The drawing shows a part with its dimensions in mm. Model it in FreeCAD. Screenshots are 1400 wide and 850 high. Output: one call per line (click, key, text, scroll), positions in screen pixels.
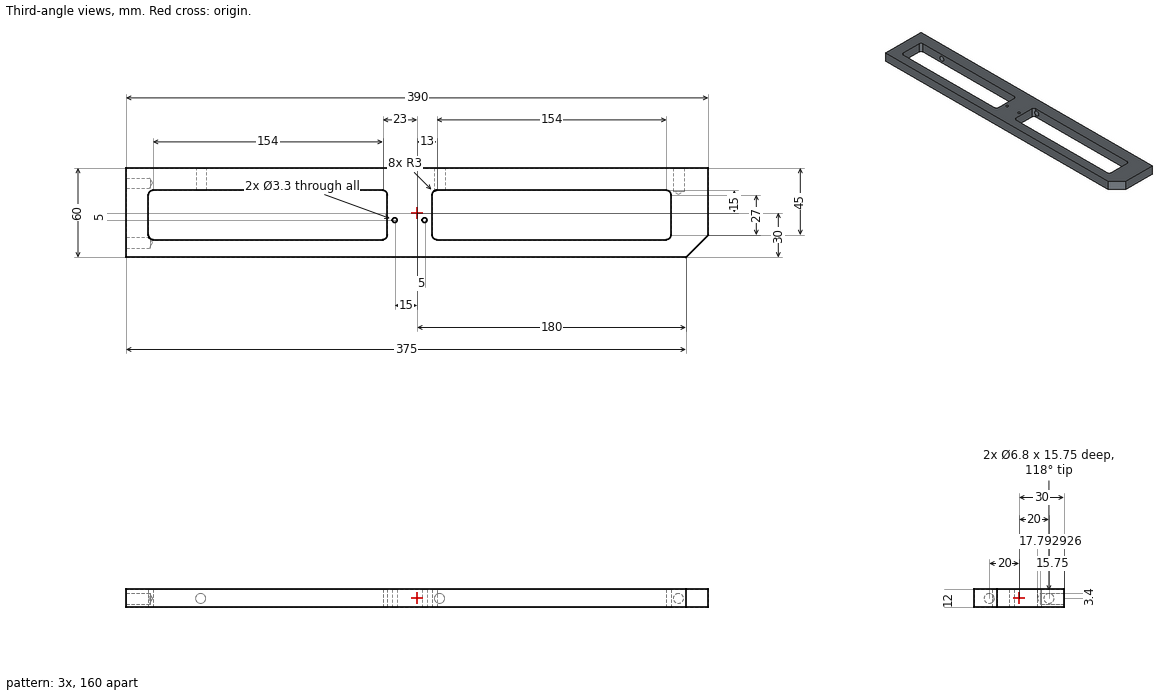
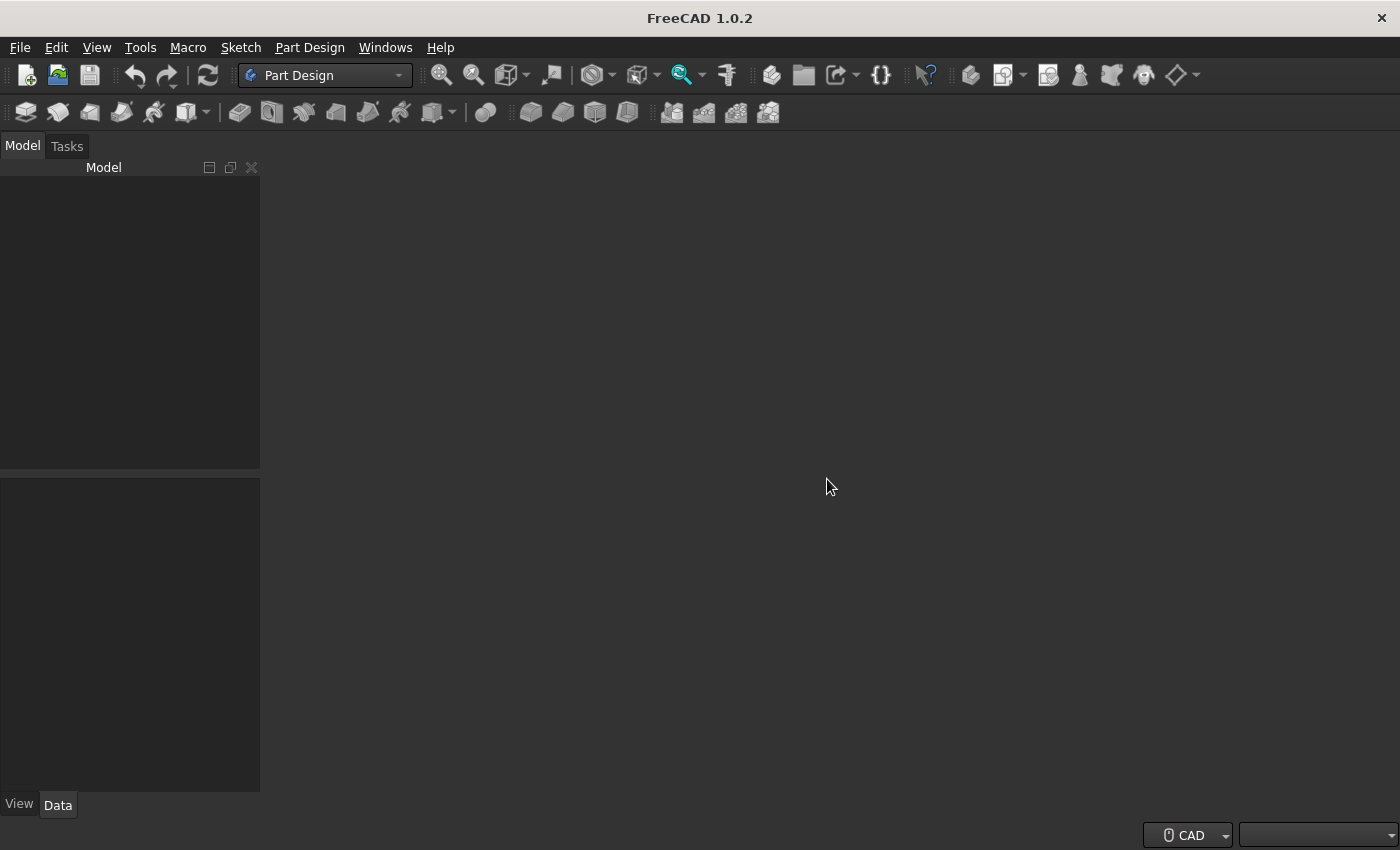
click(26, 76)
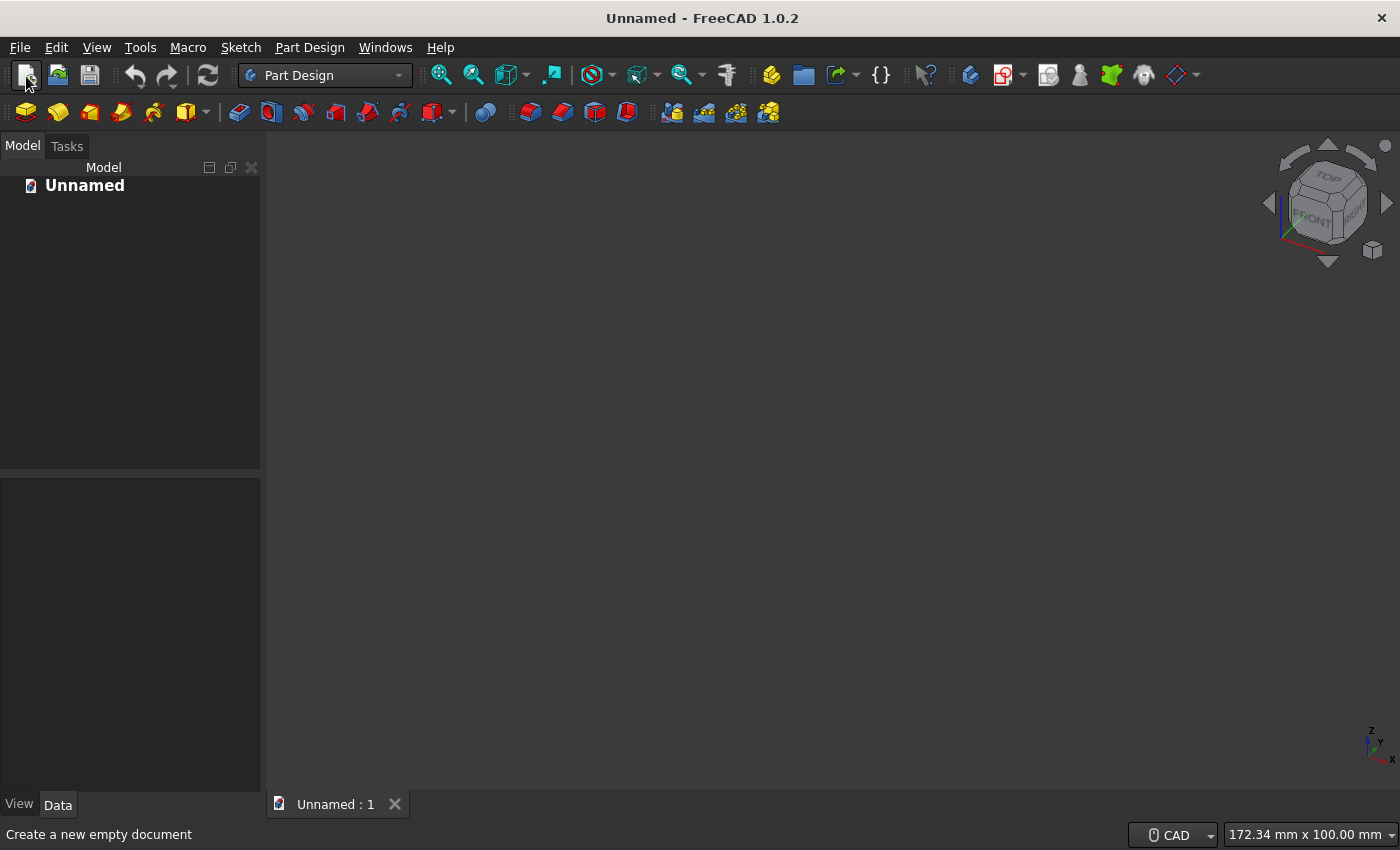
click(1004, 76)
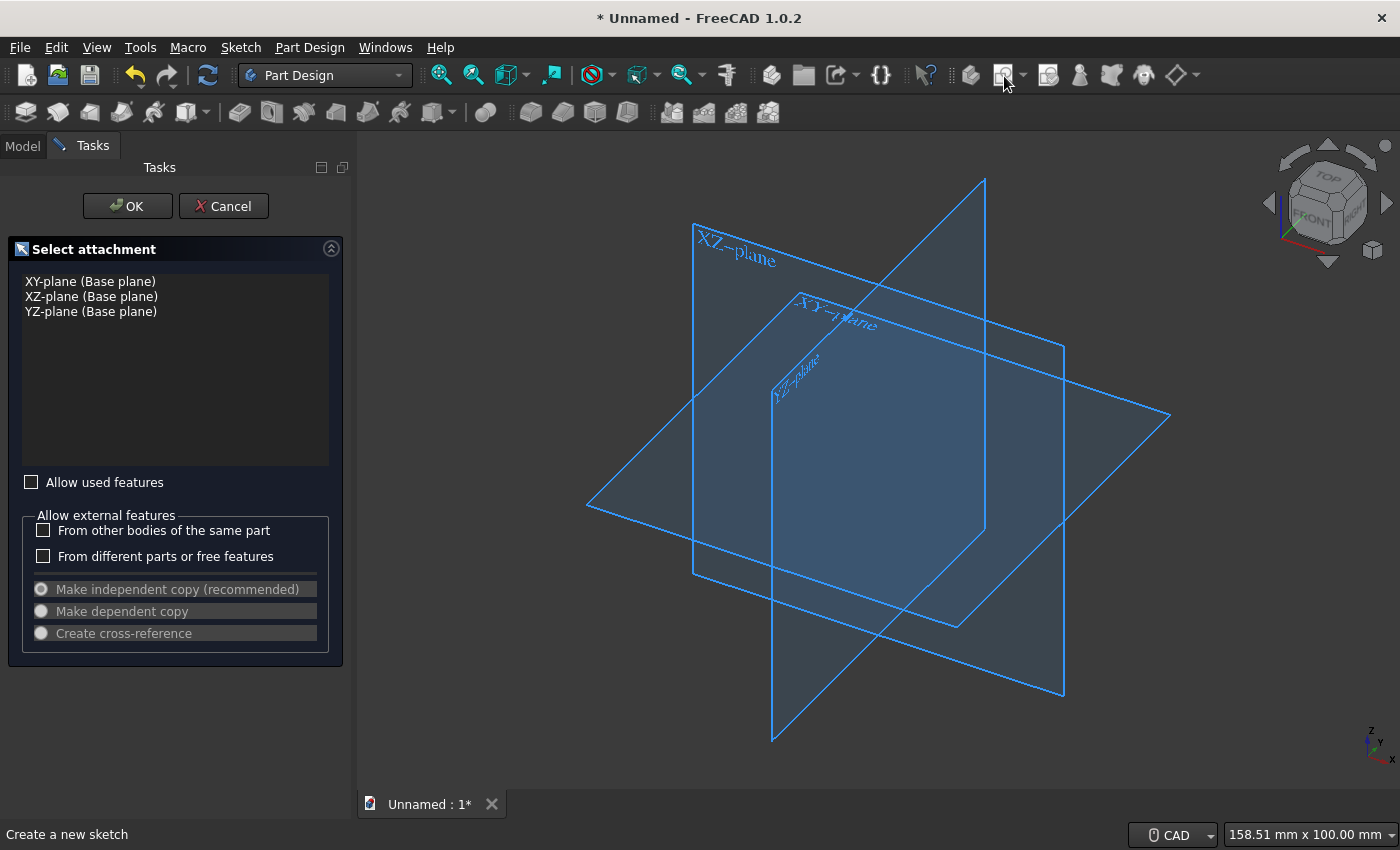
click(82, 282)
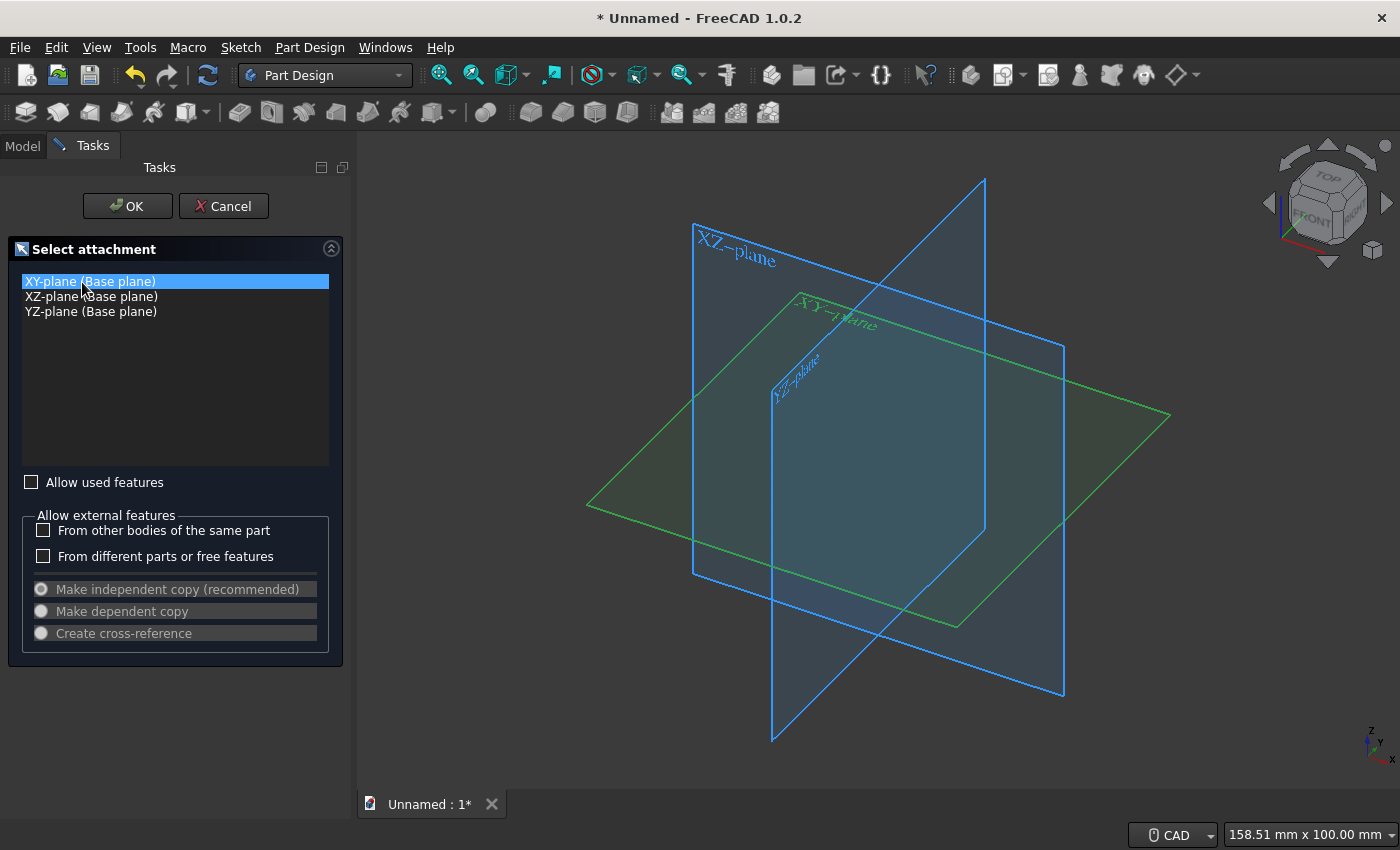
click(128, 206)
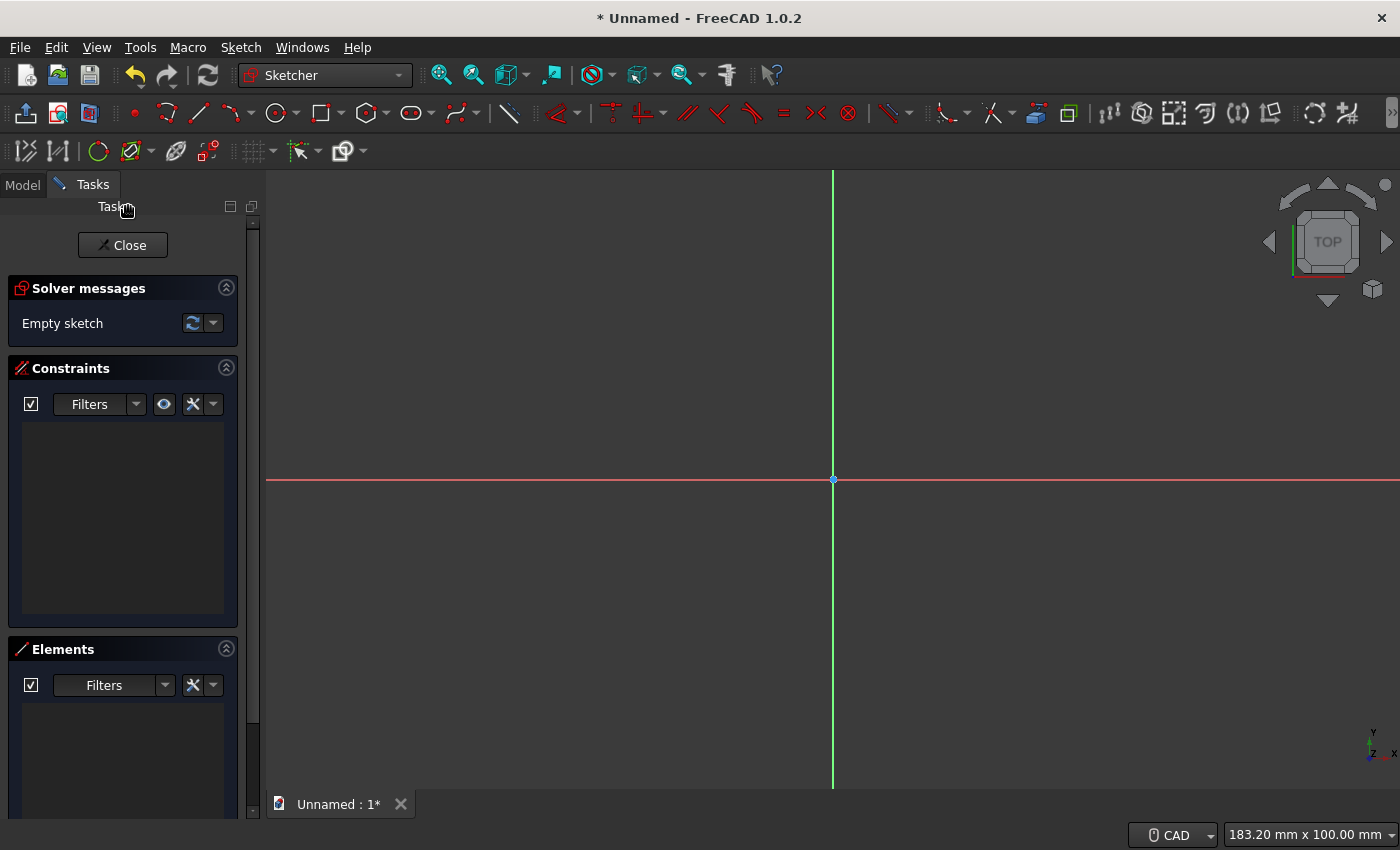
scroll(735, 480, down, 6)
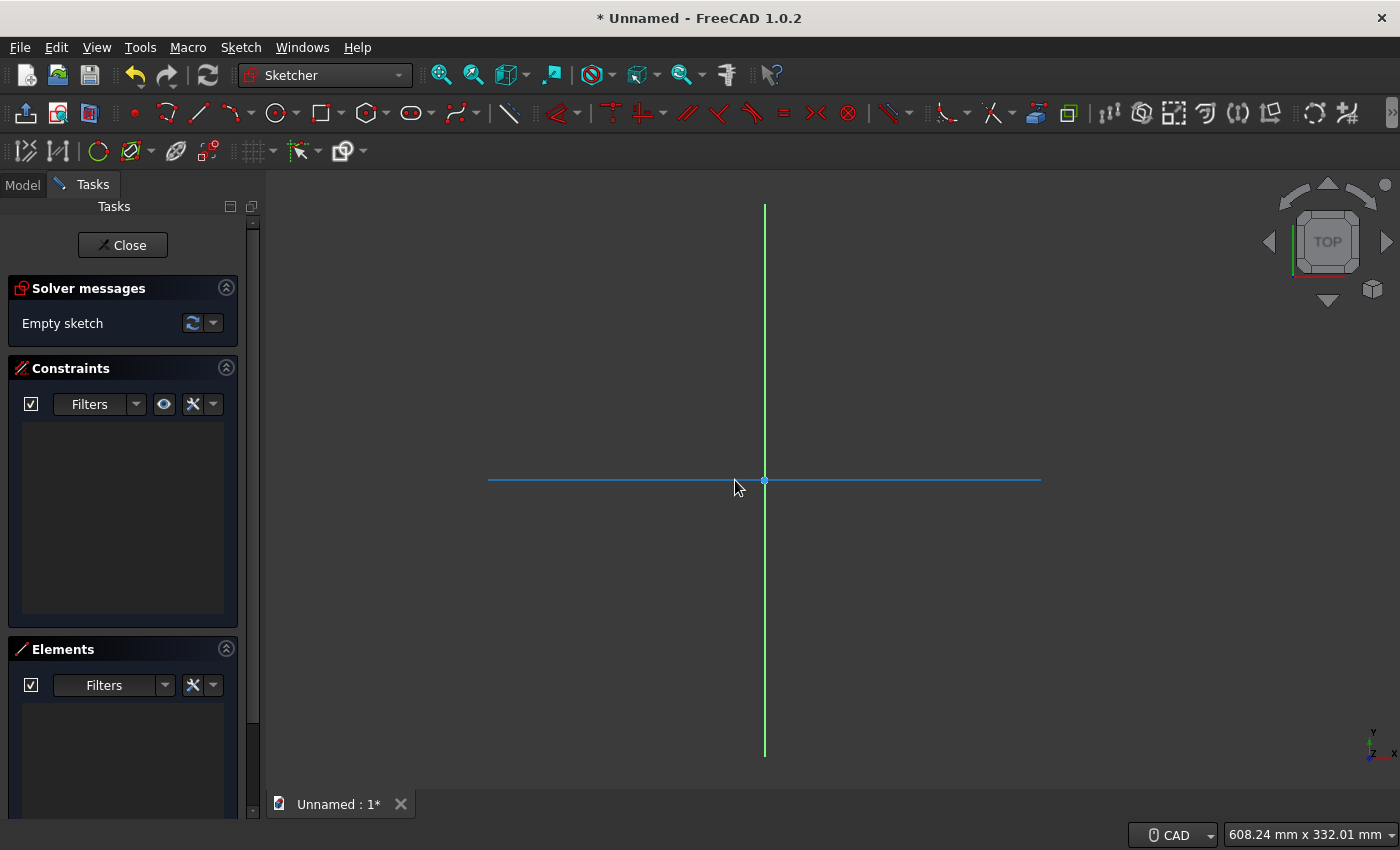
key(g)
key(m)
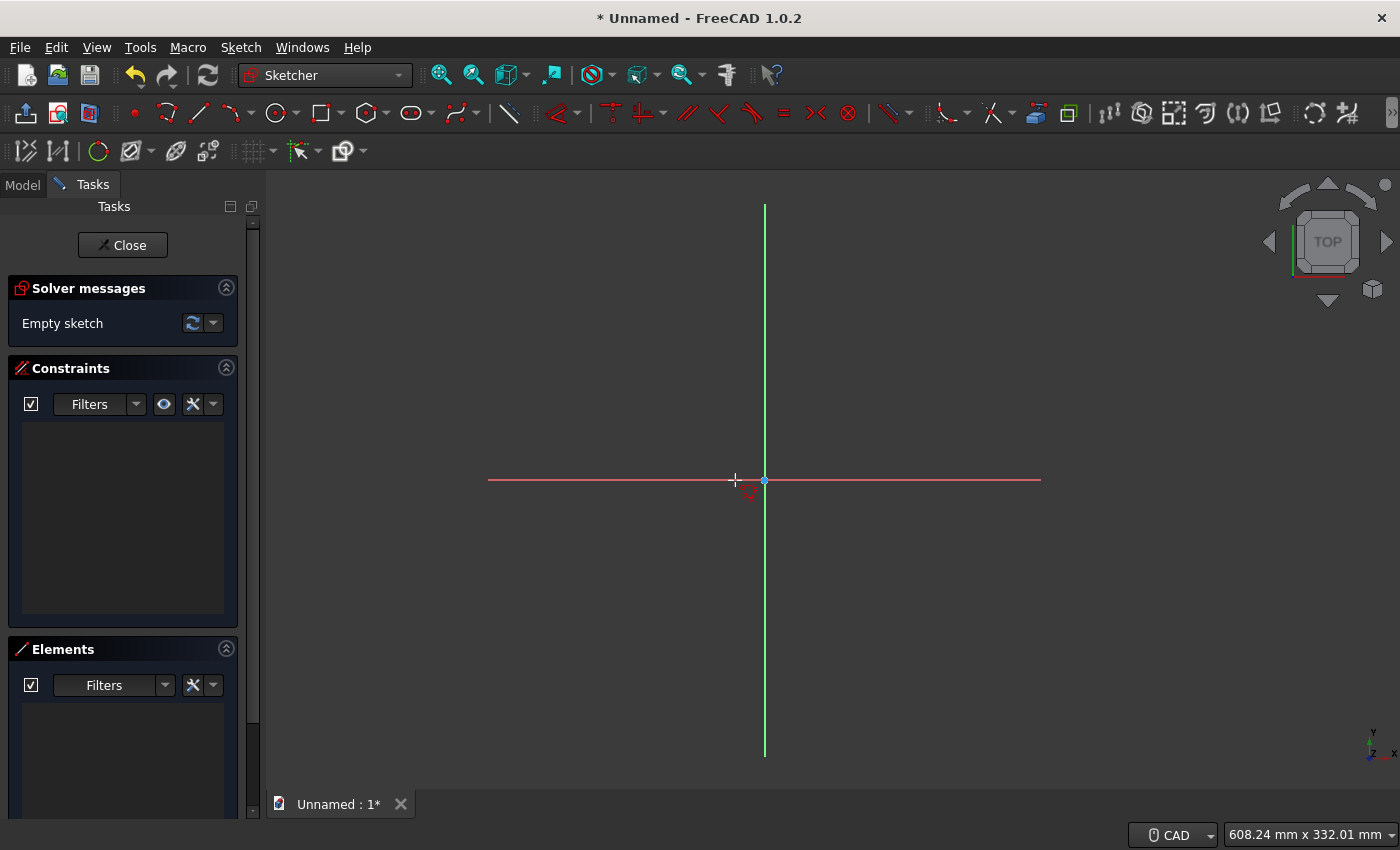
click(1100, 536)
click(1128, 508)
click(1128, 424)
click(401, 424)
click(401, 536)
click(1100, 537)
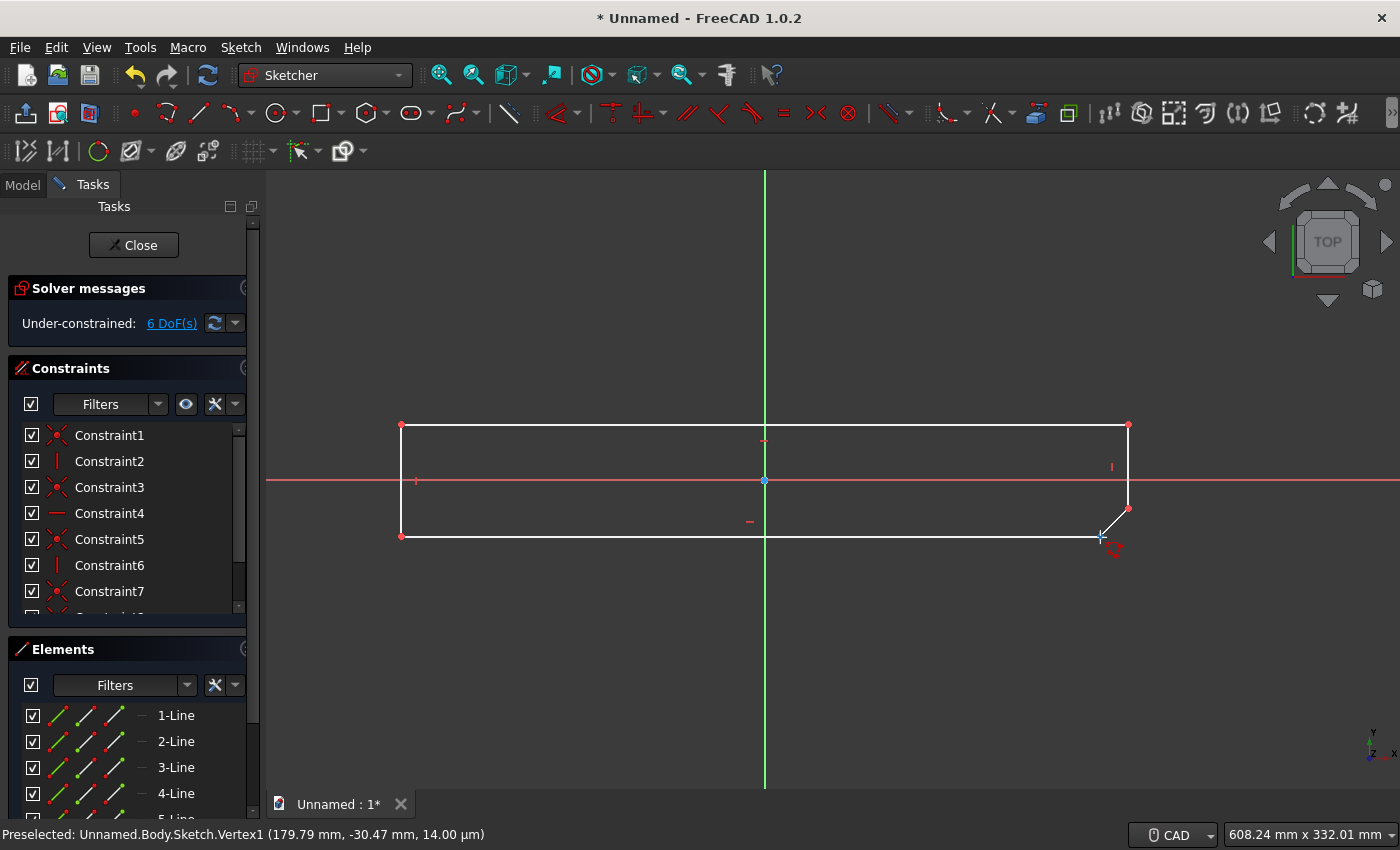
click(200, 114)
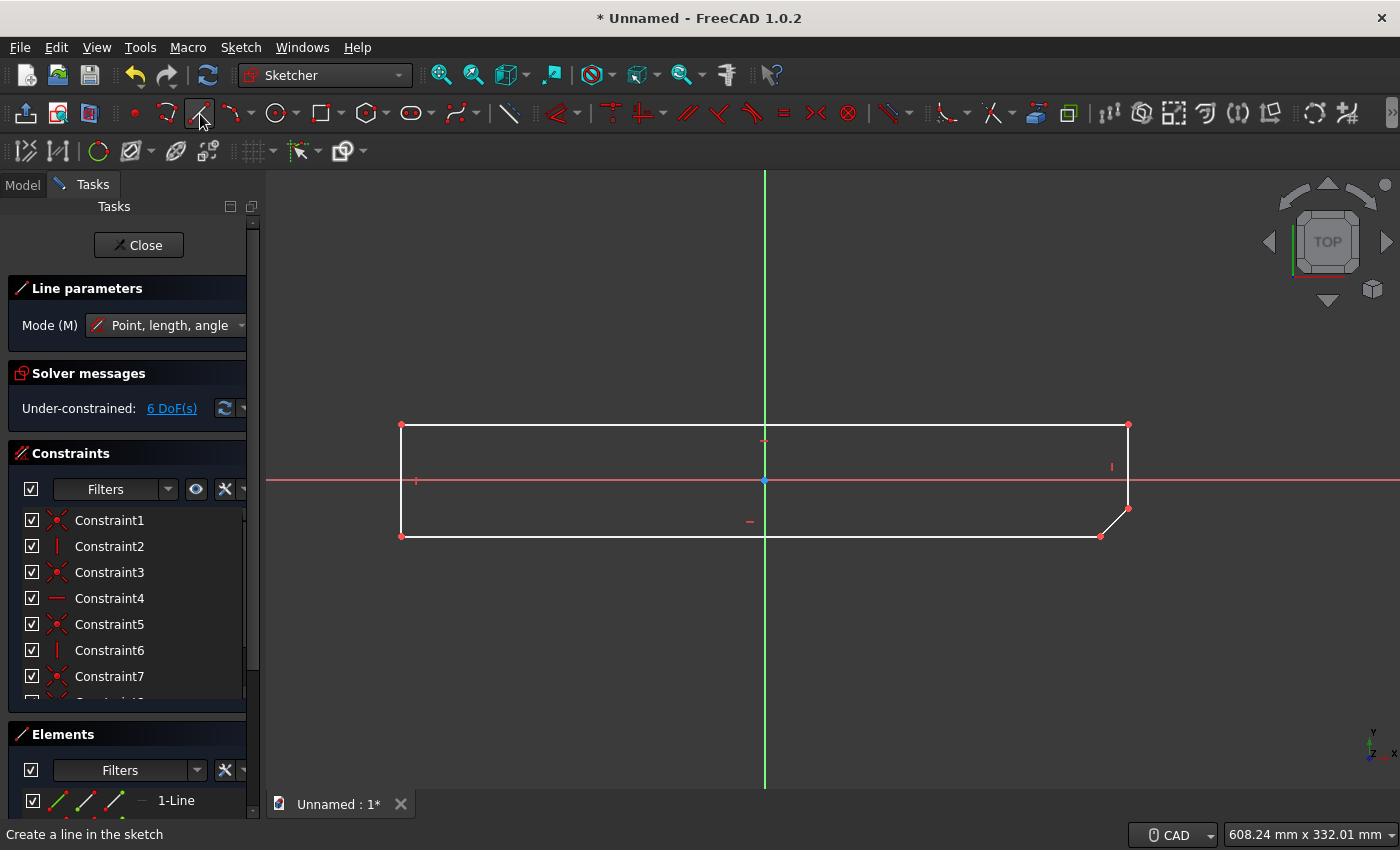
click(789, 452)
click(1076, 452)